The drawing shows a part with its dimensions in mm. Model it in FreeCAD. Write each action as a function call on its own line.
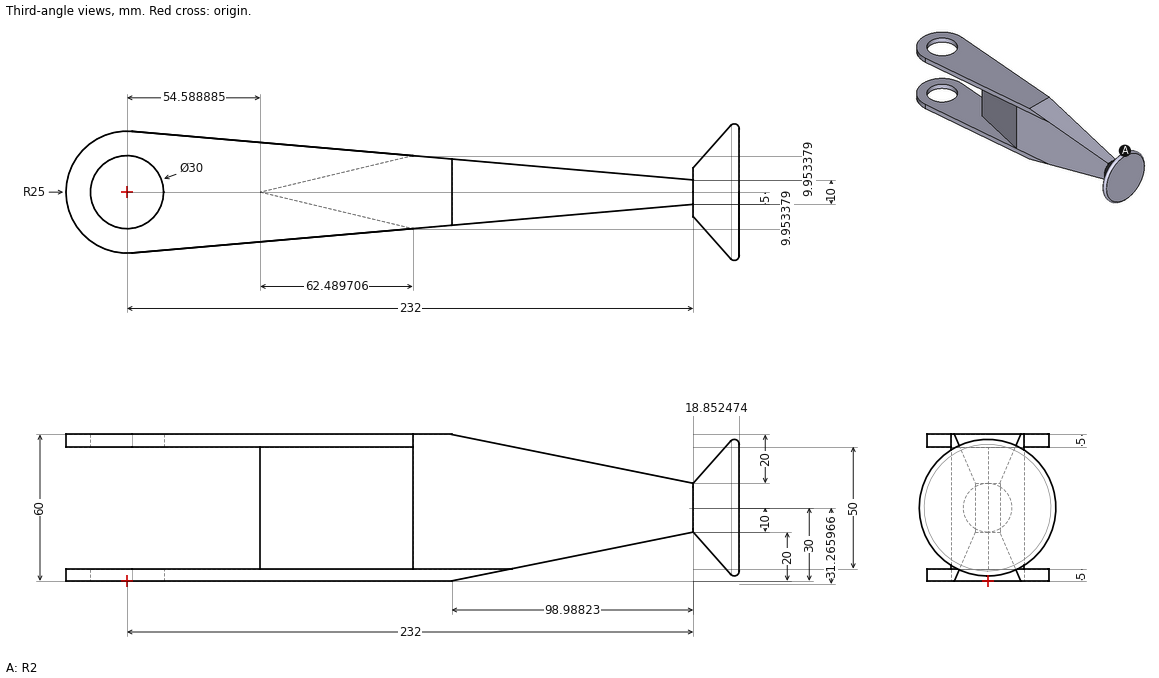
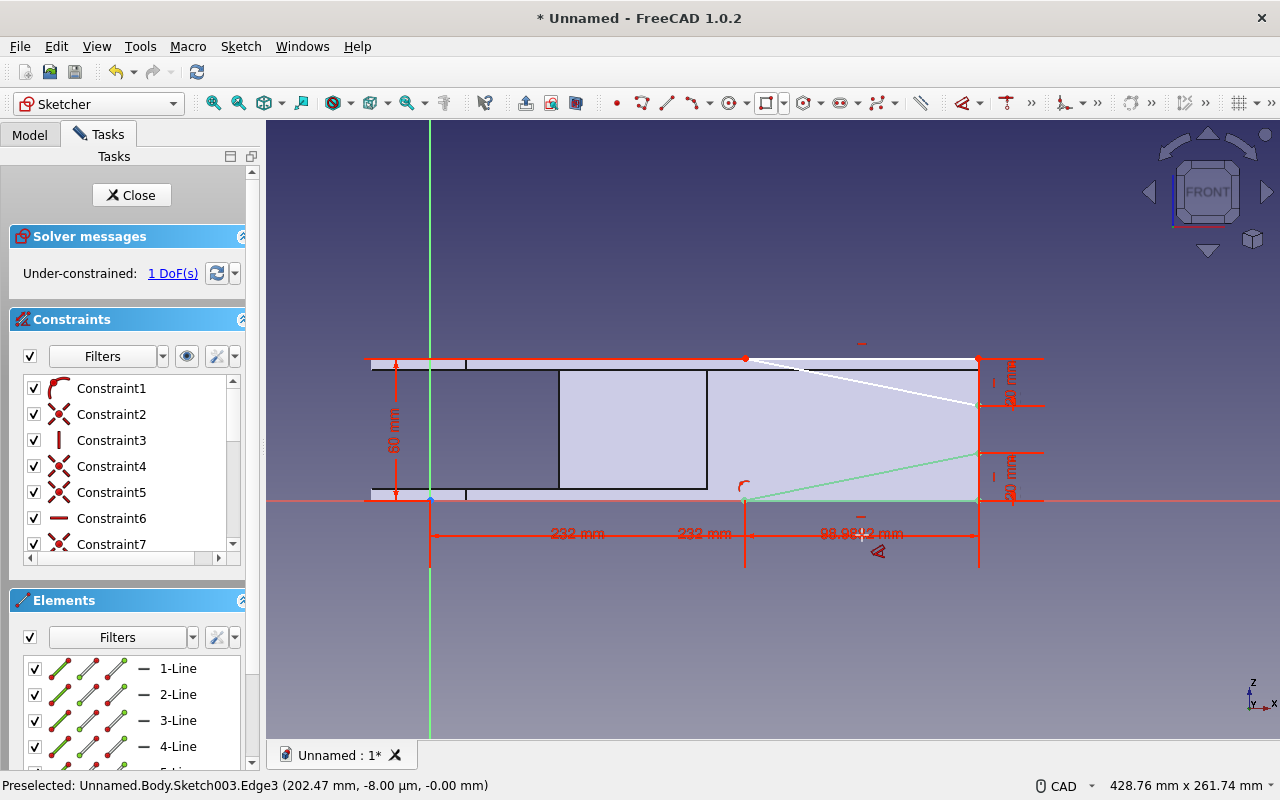
click(815, 359)
click(862, 325)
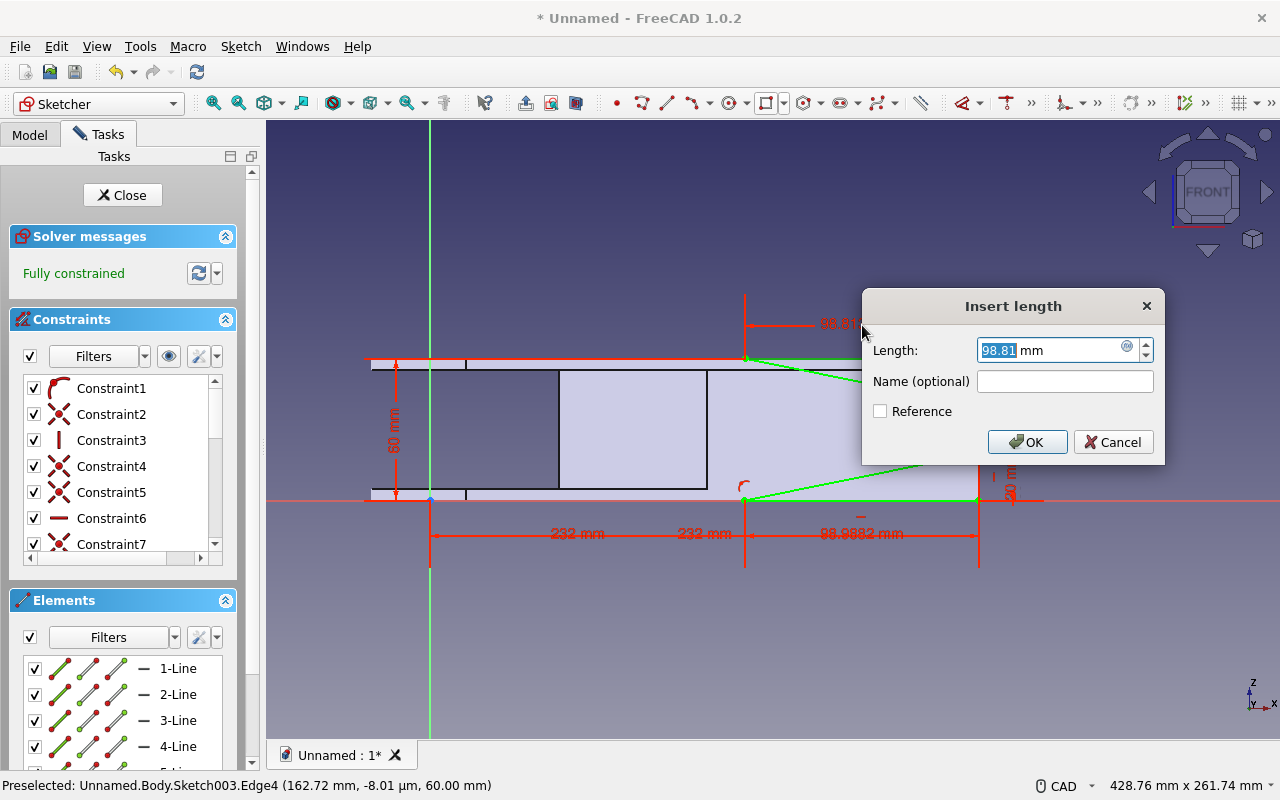
text(98.98823)
key(Return)
key(Escape)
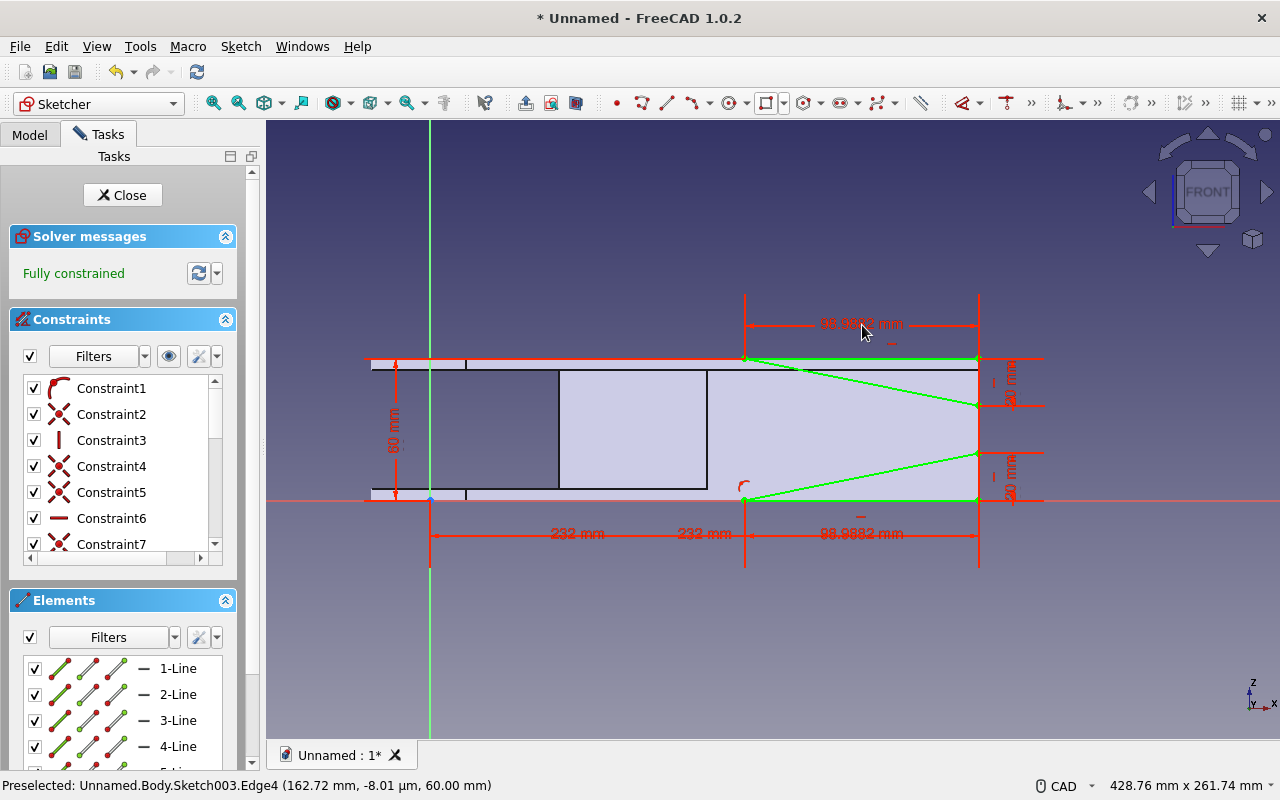
click(123, 195)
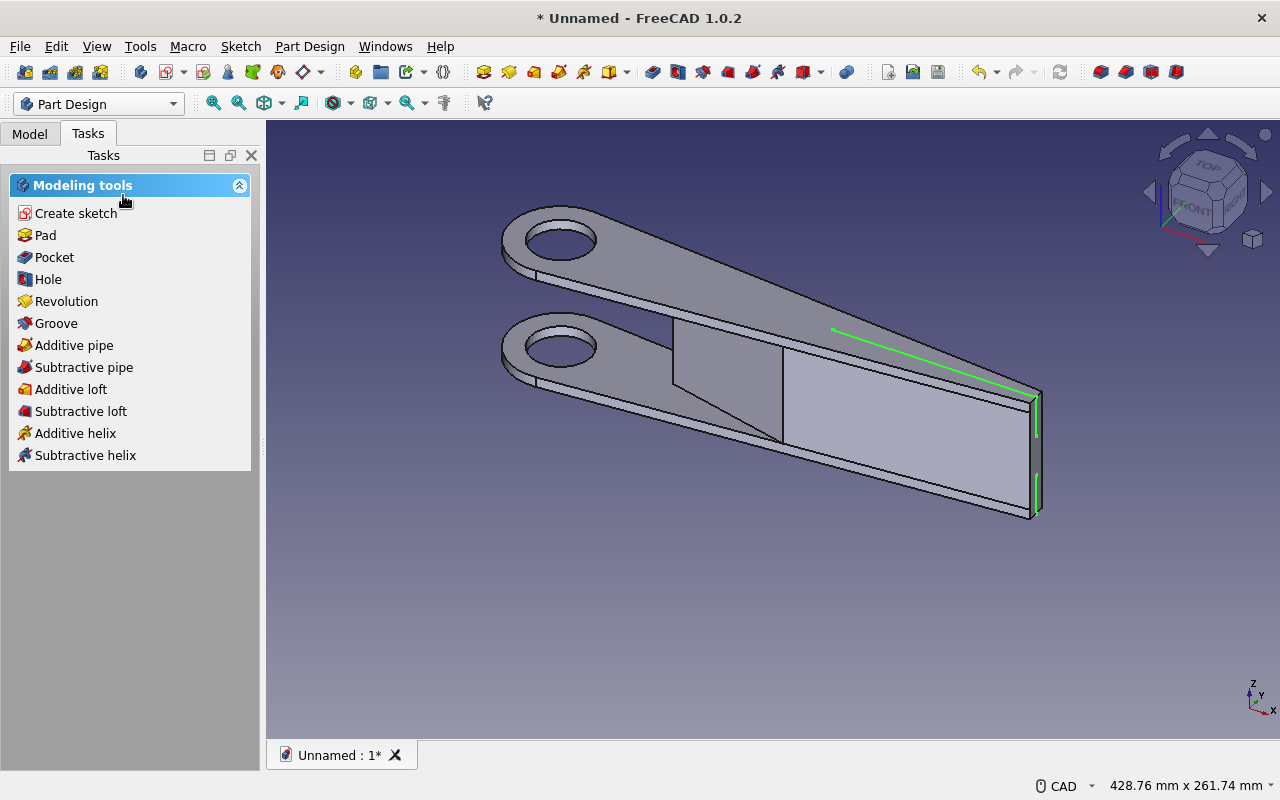
click(653, 72)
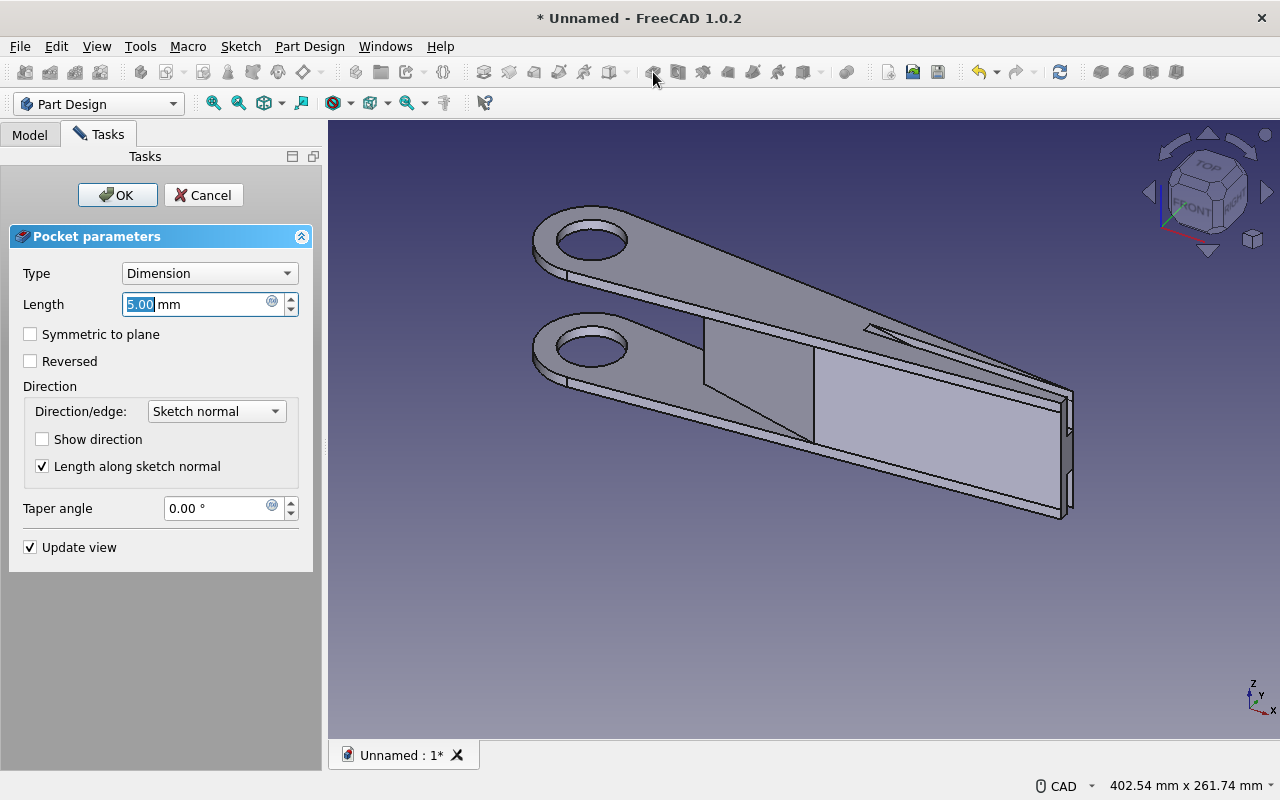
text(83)
key(Tab)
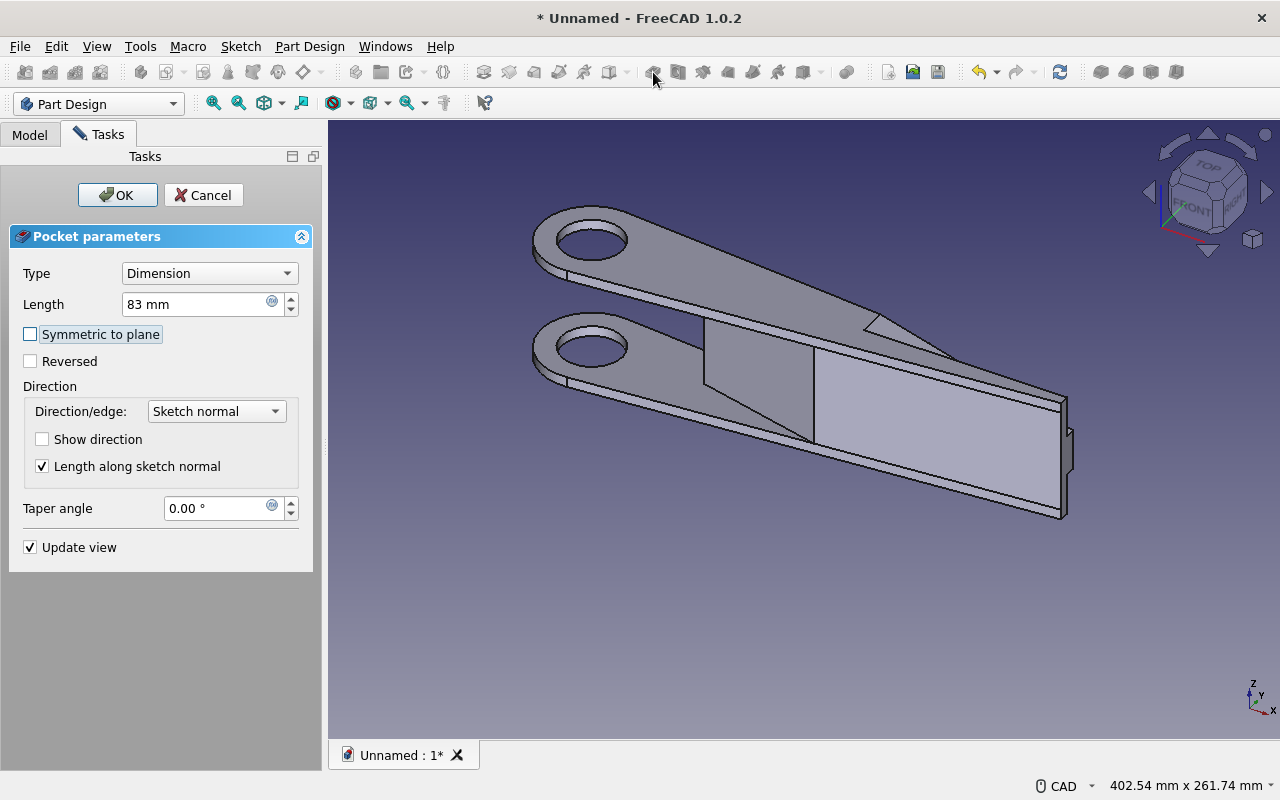
click(31, 334)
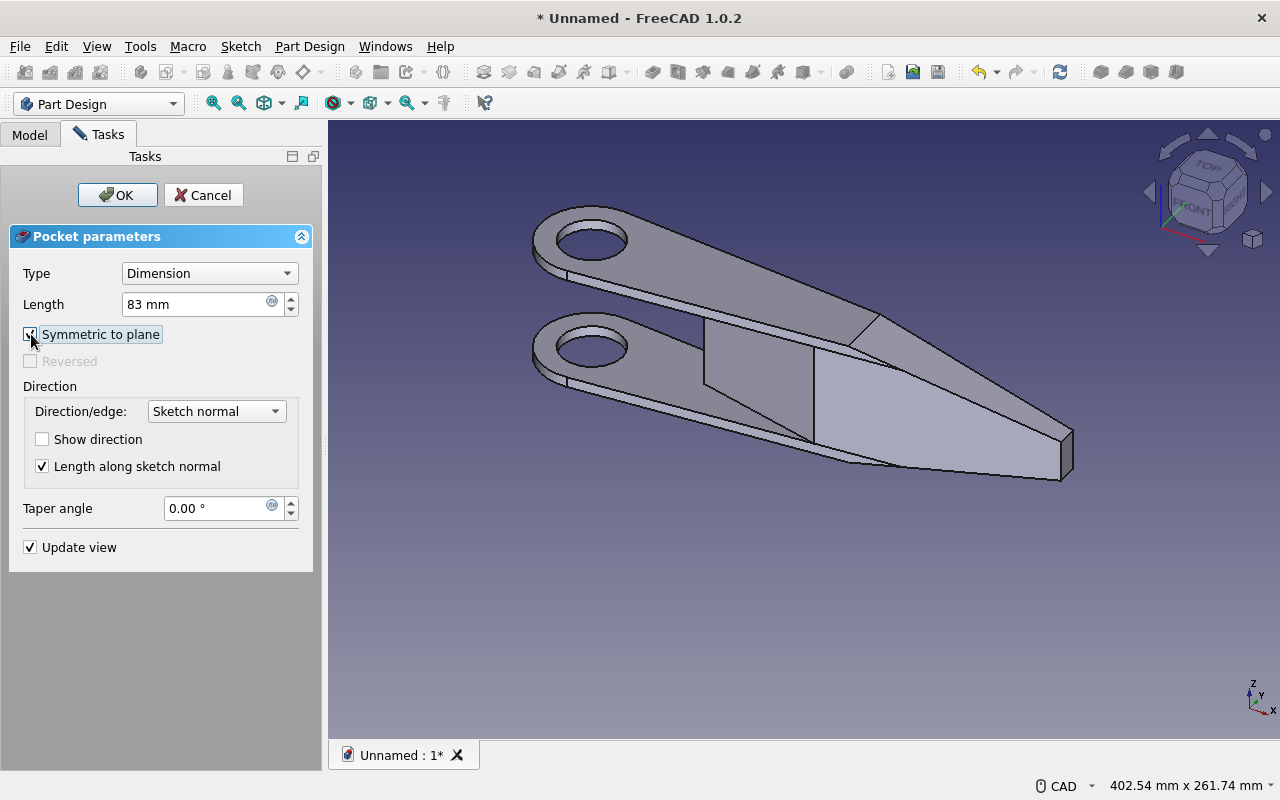
click(118, 195)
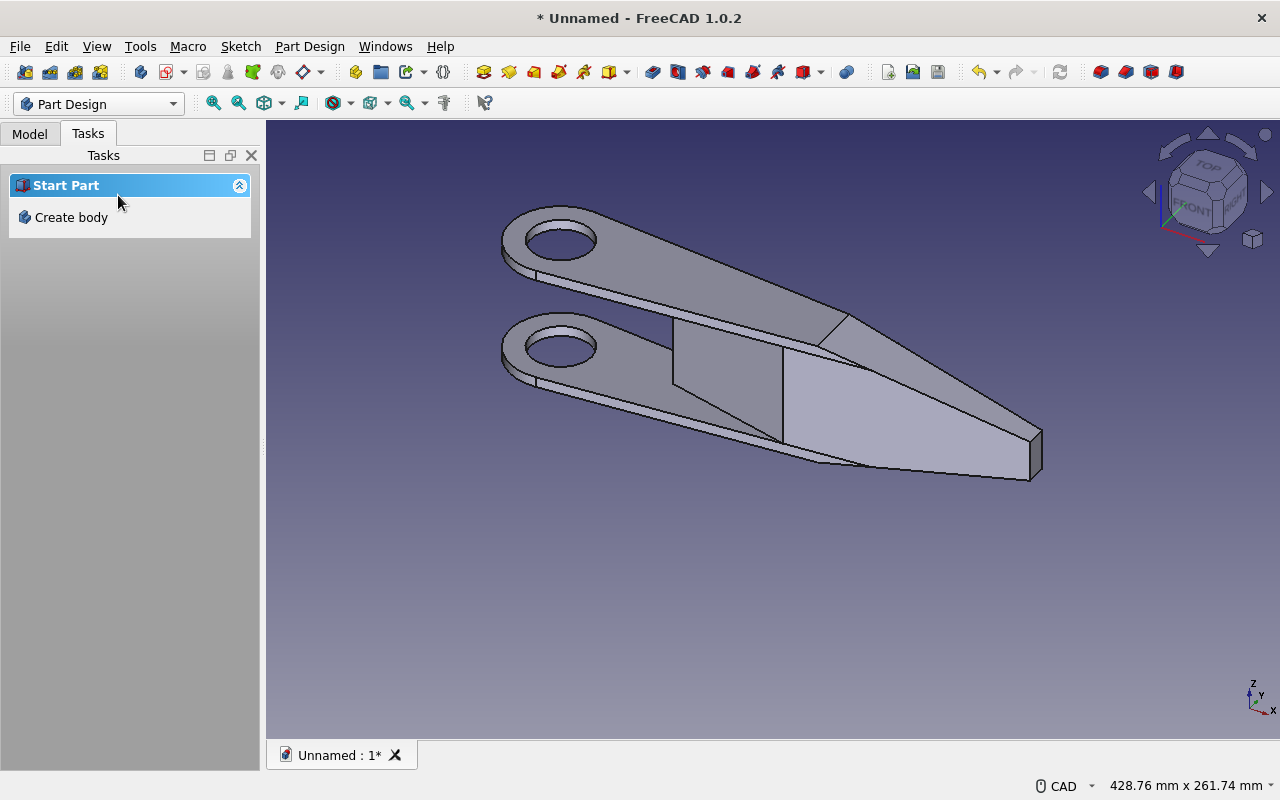
click(166, 72)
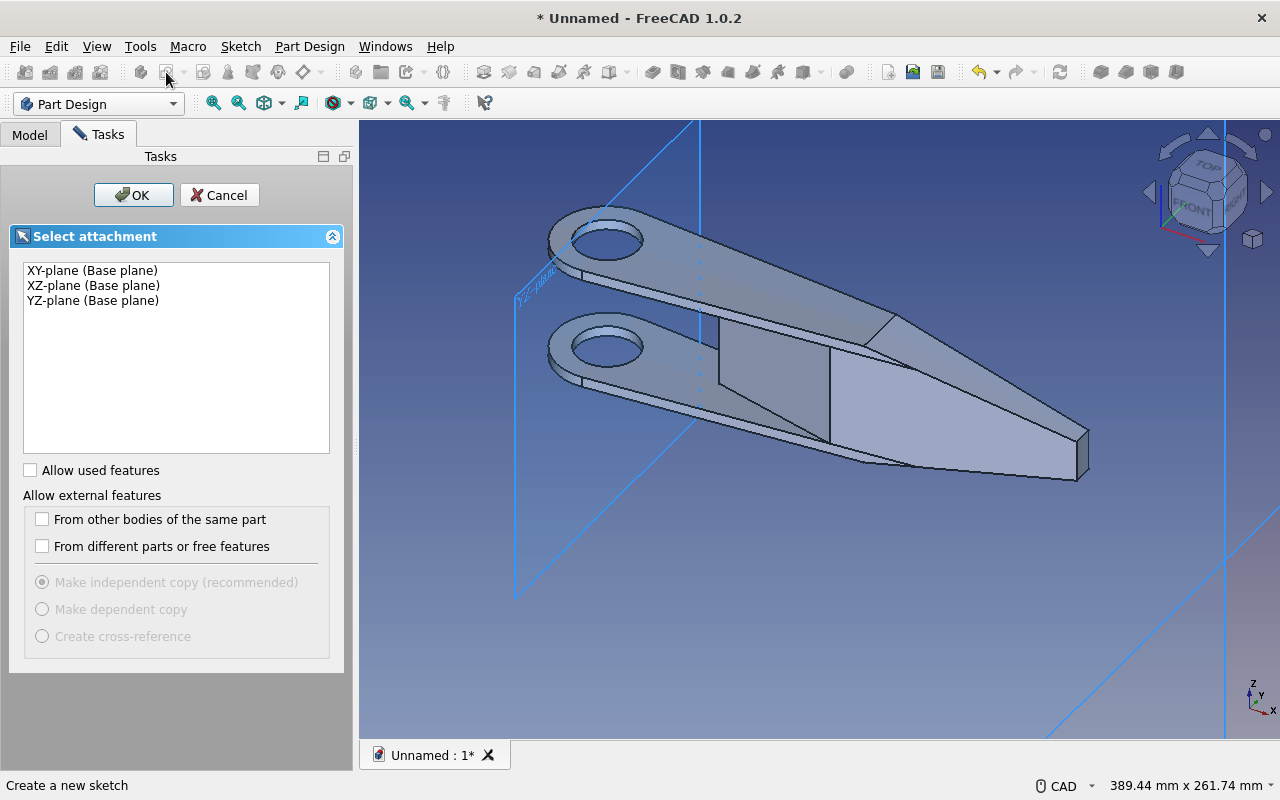
click(84, 286)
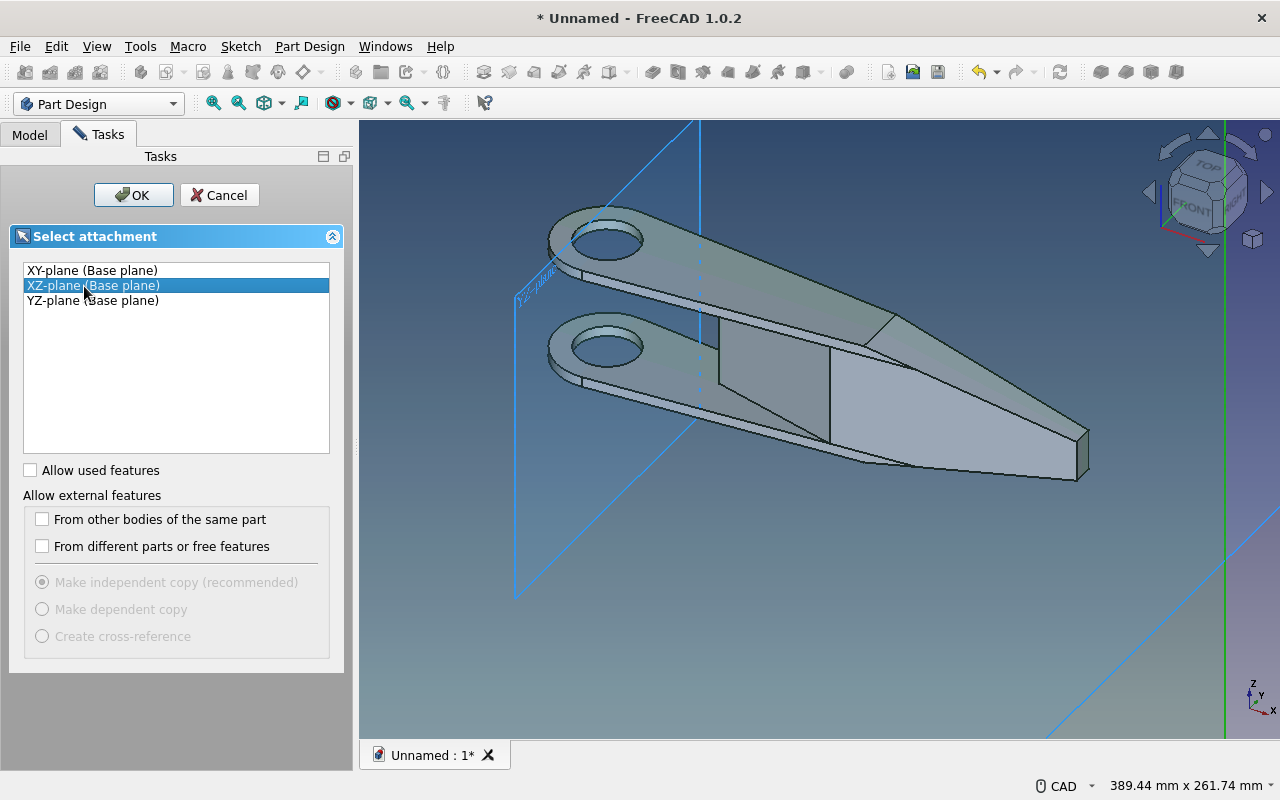
click(134, 195)